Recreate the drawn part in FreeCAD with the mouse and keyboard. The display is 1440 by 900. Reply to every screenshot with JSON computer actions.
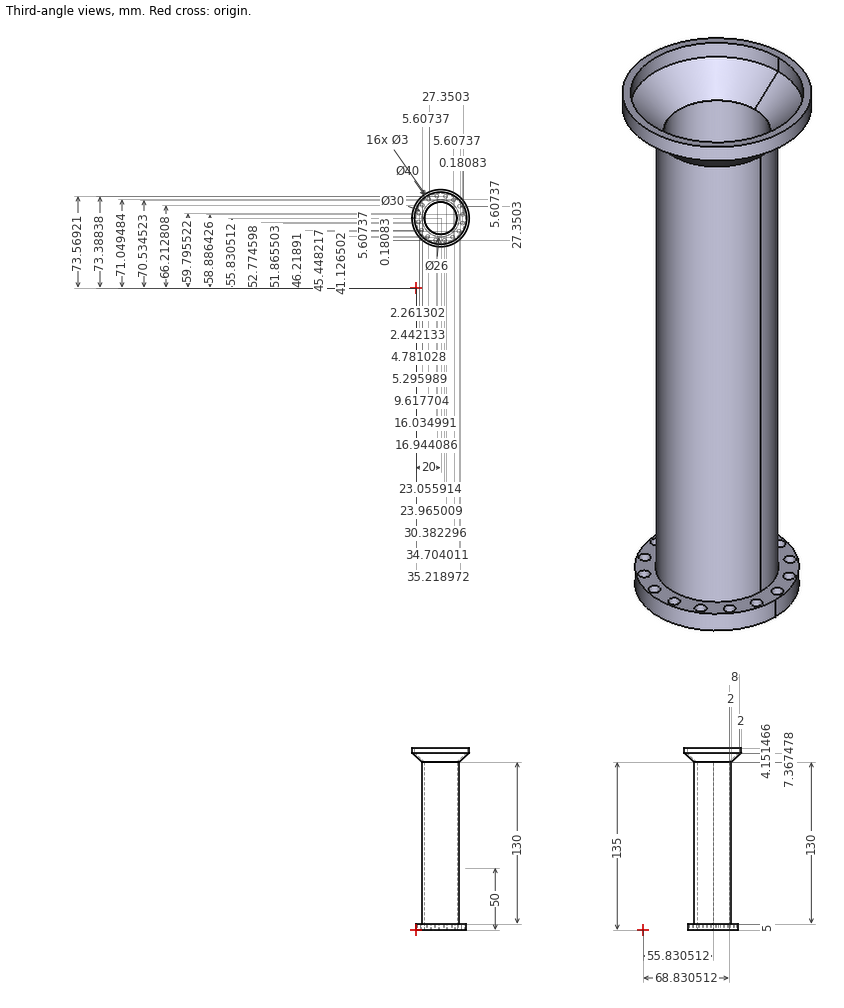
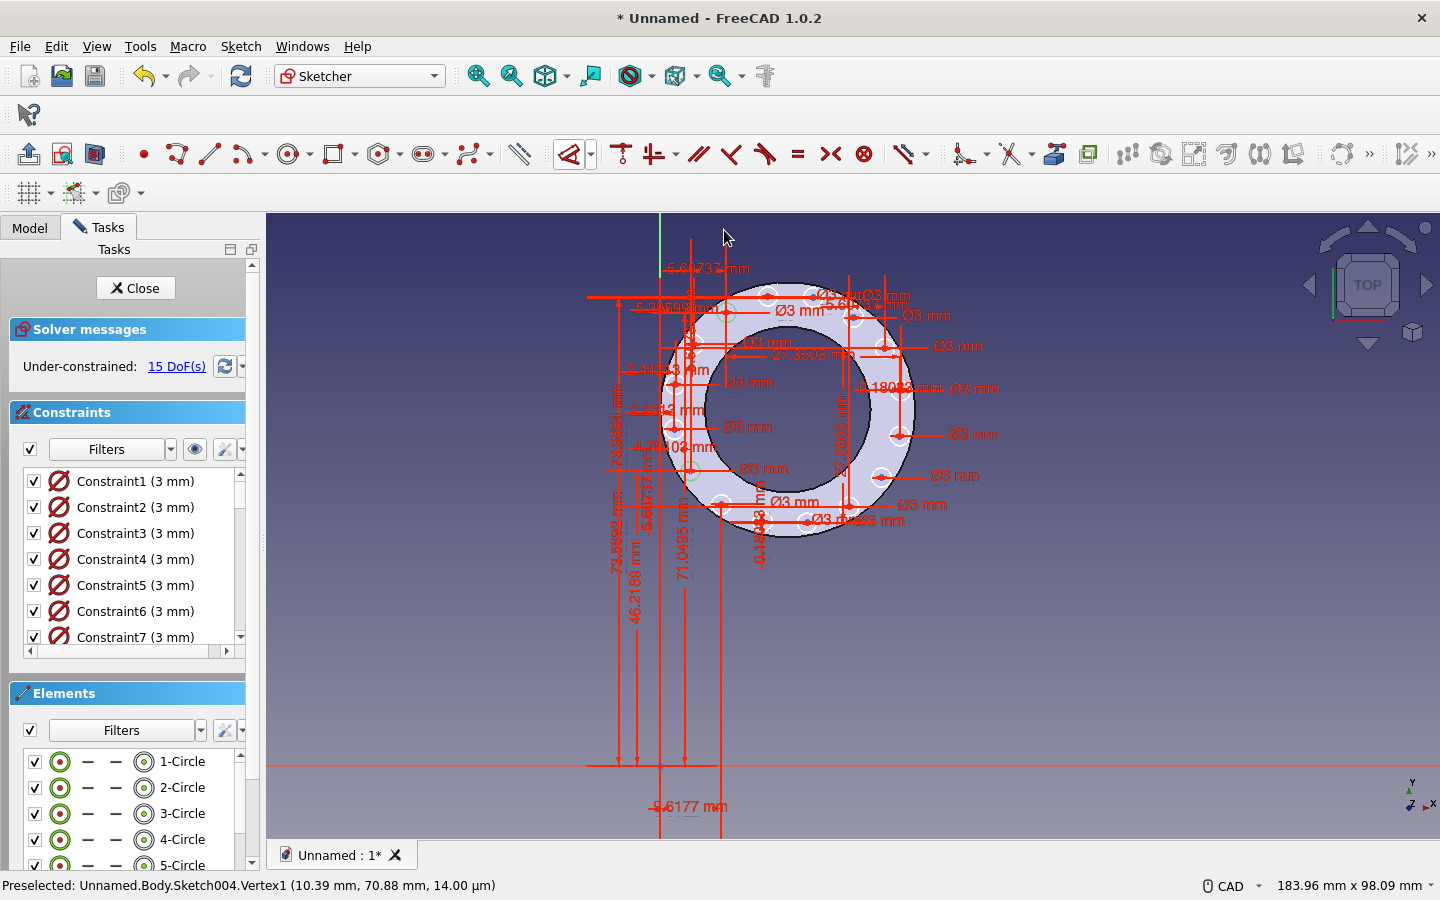
{"action": "left_click", "coordinate": [768, 297]}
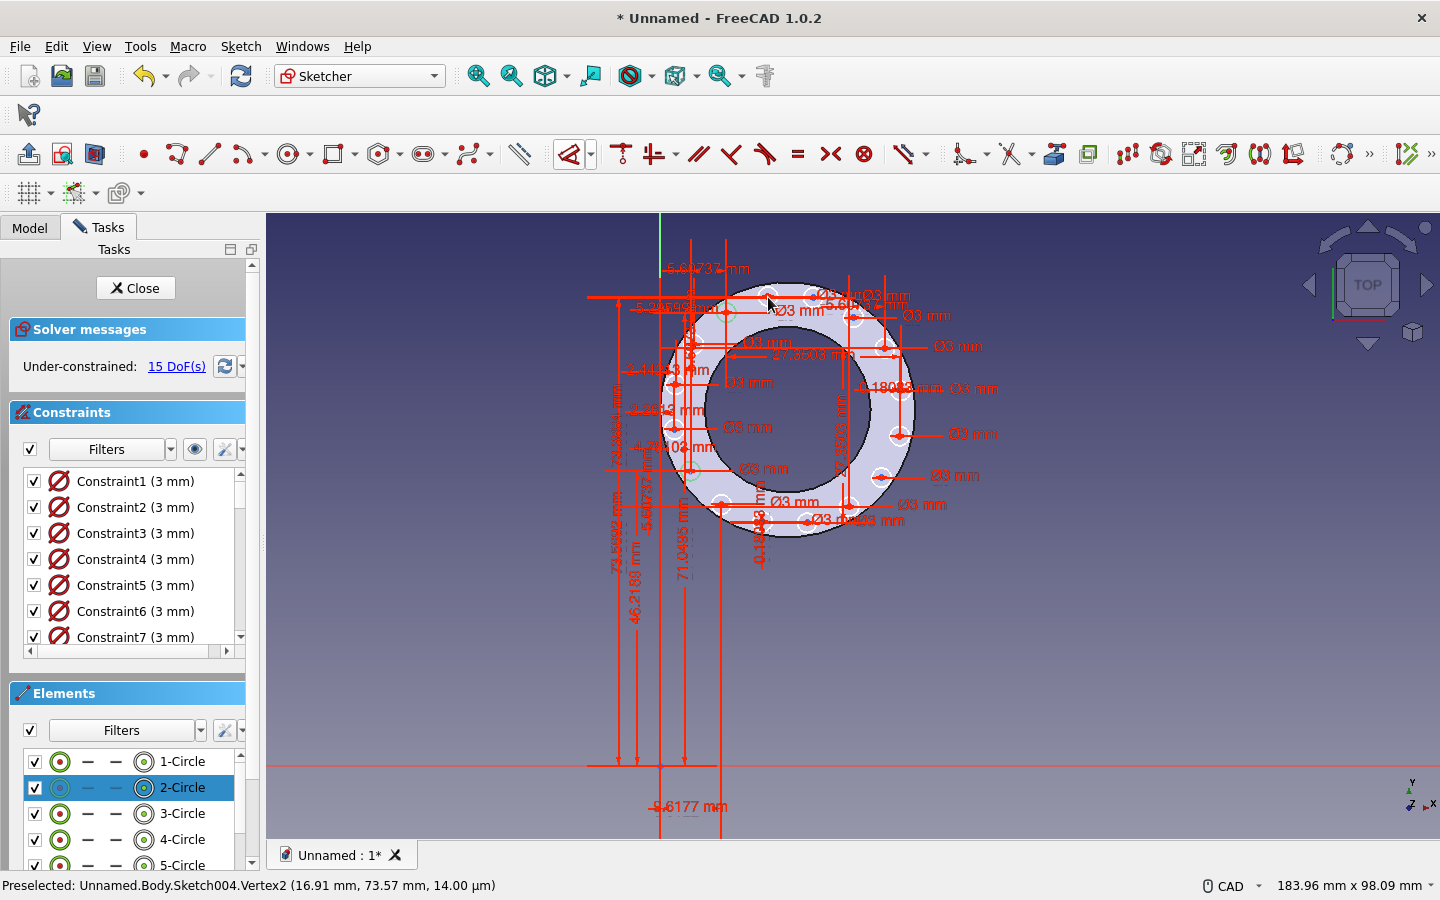
{"action": "left_click", "coordinate": [590, 154]}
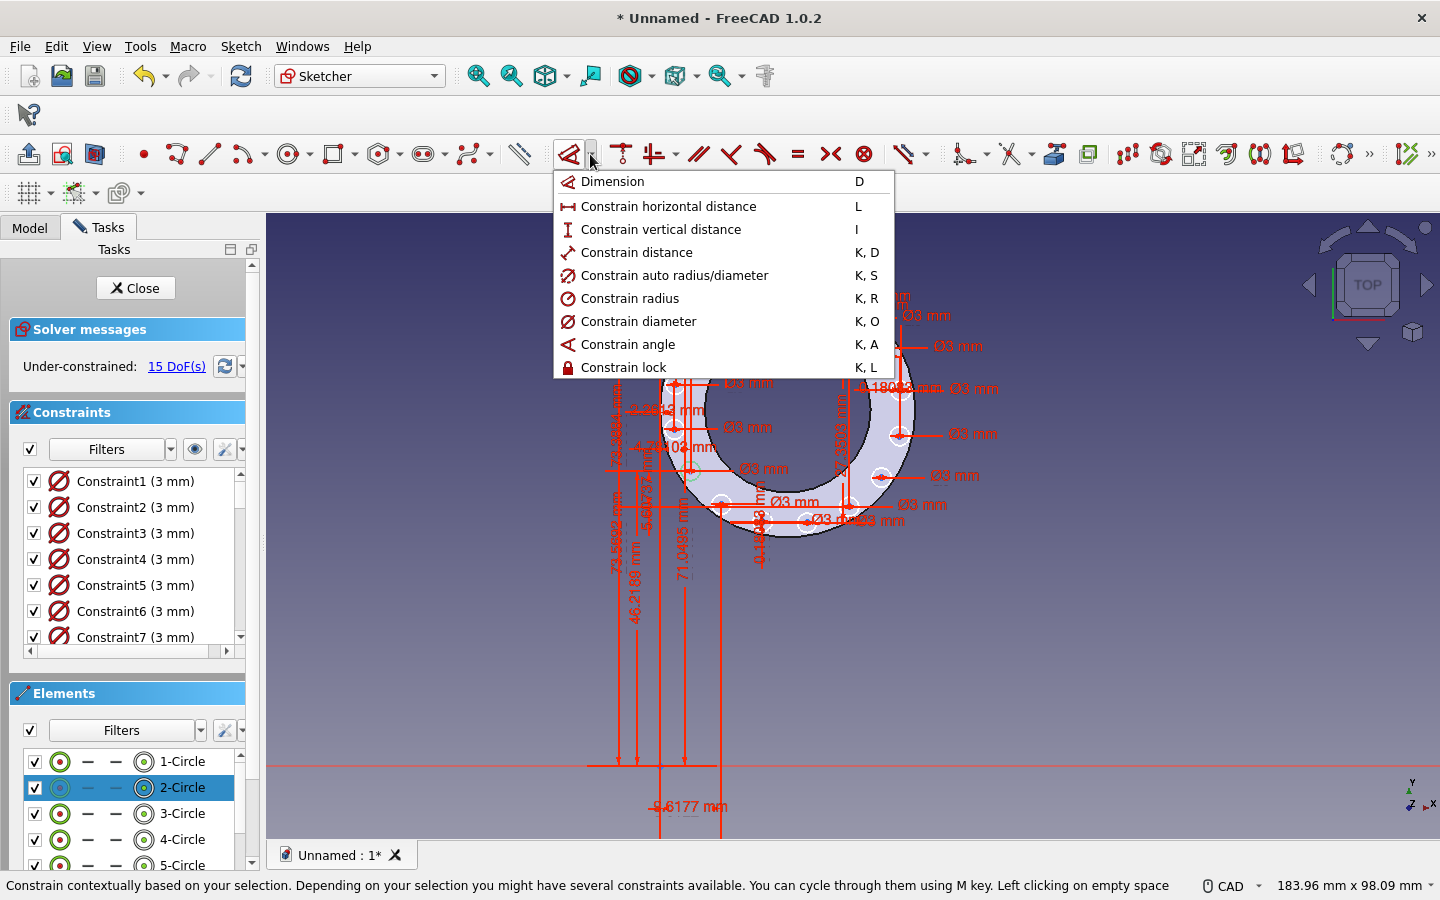
{"action": "left_click", "coordinate": [724, 206]}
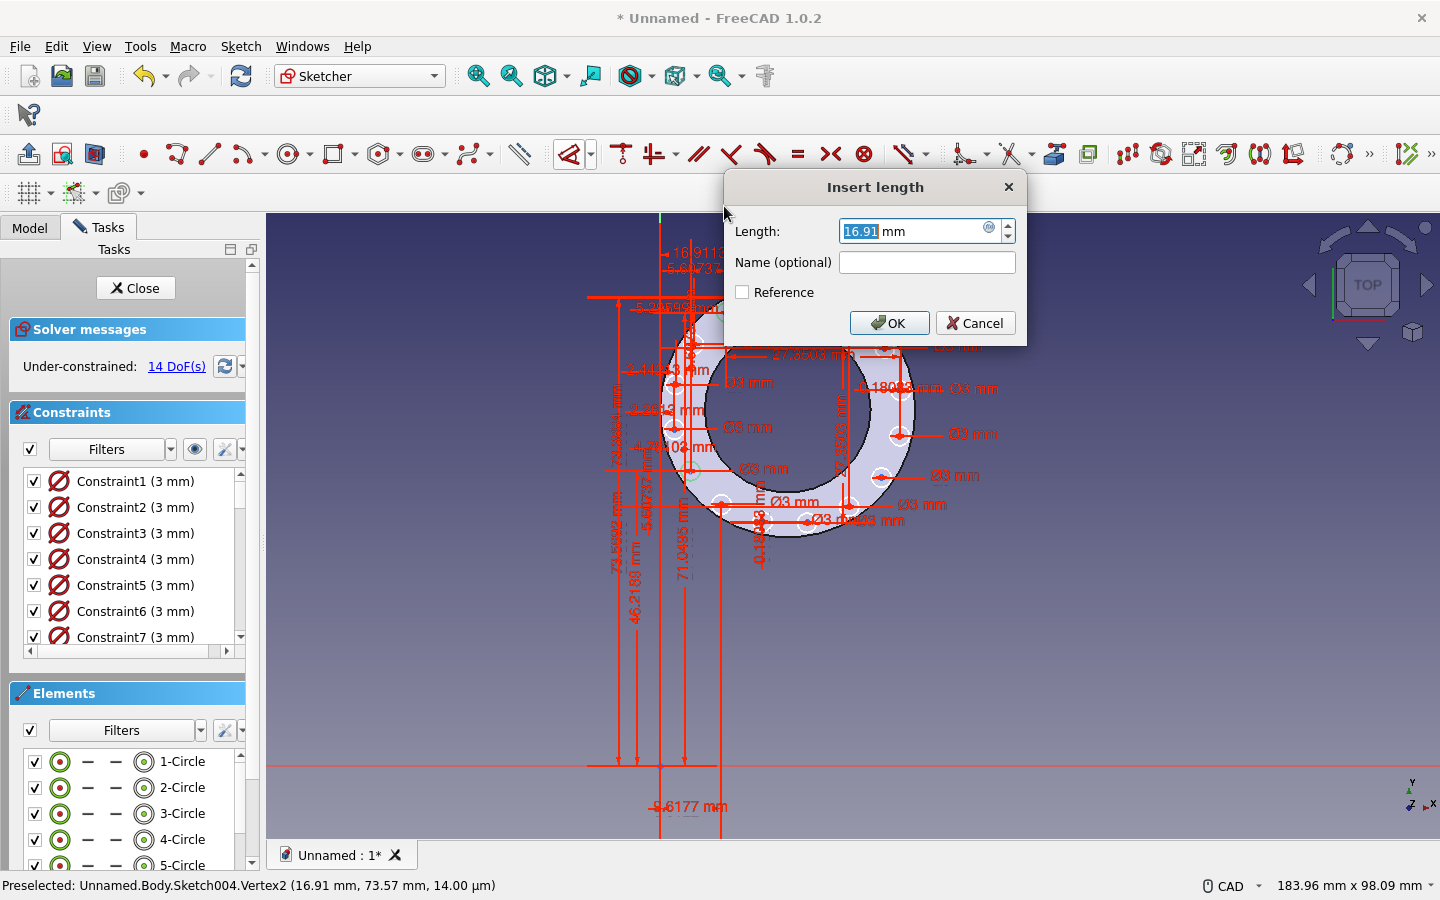
{"action": "type", "text": "16.944086"}
{"action": "key", "text": "Return"}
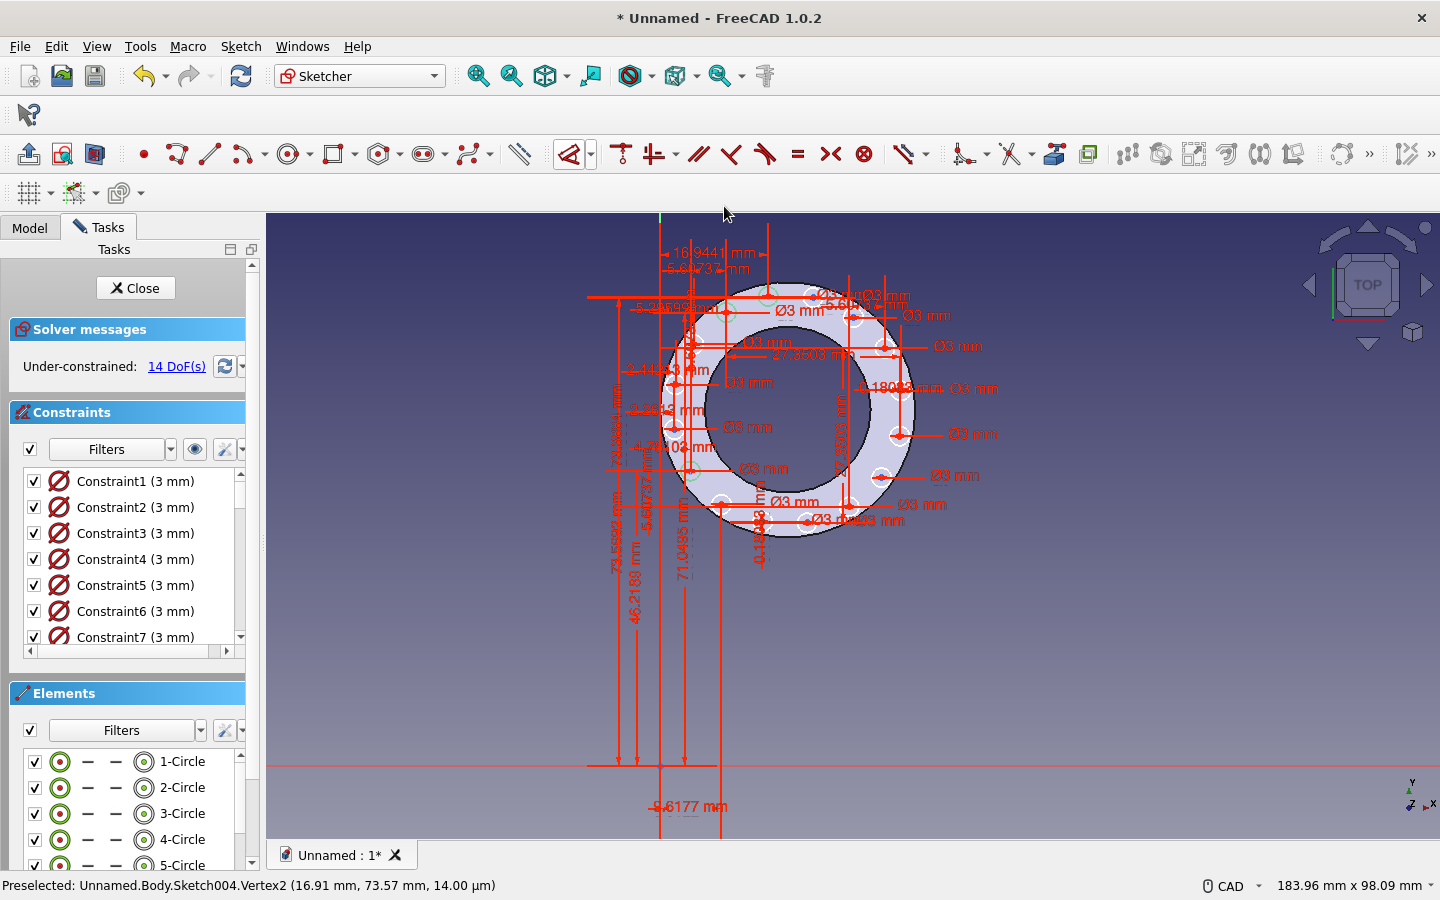
{"action": "left_click", "coordinate": [813, 298]}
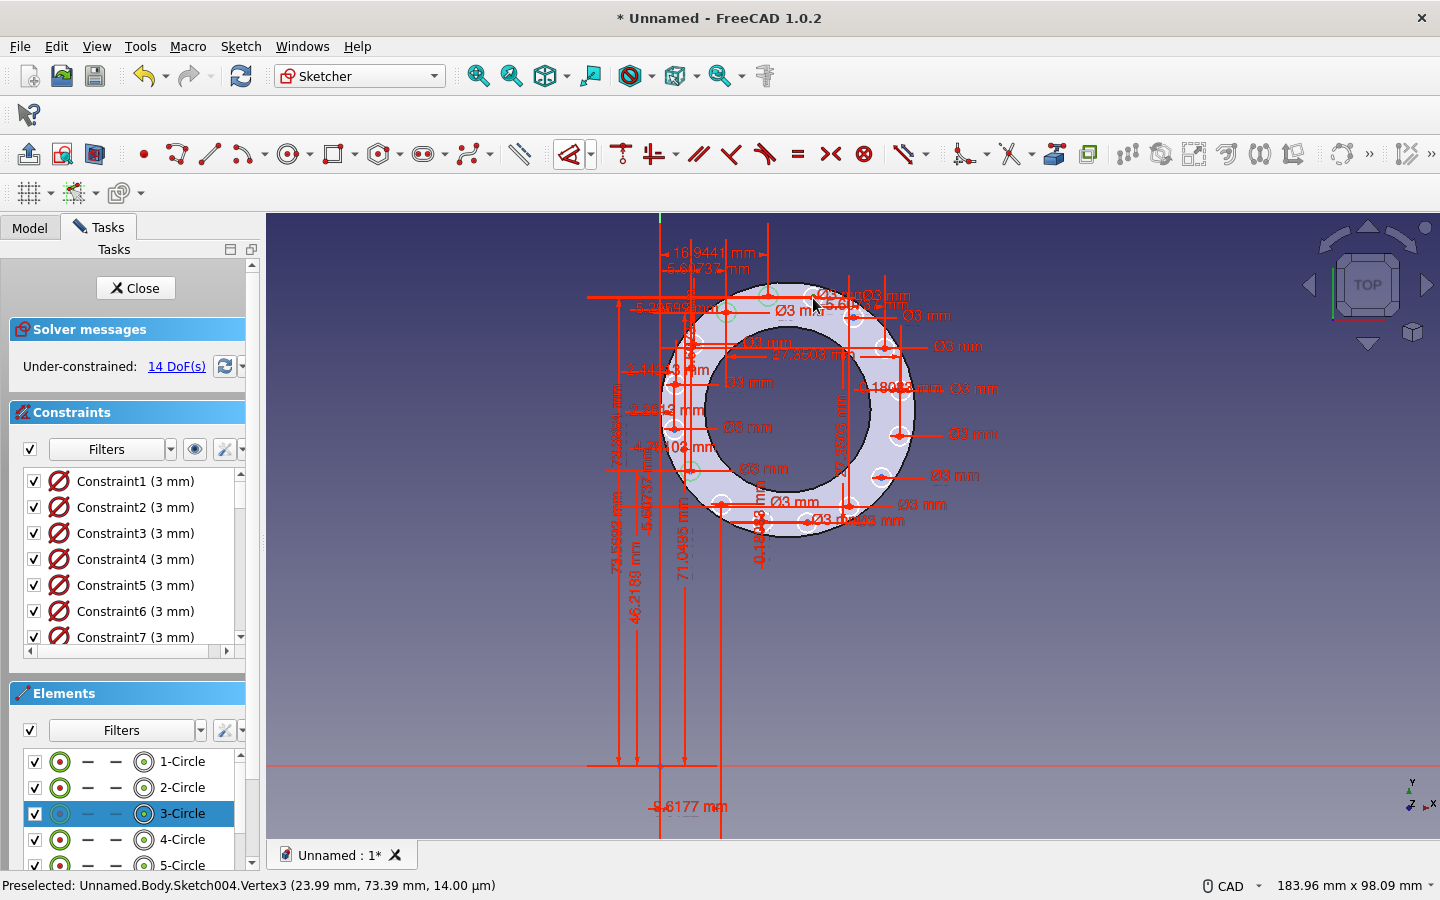
{"action": "left_click", "coordinate": [590, 154]}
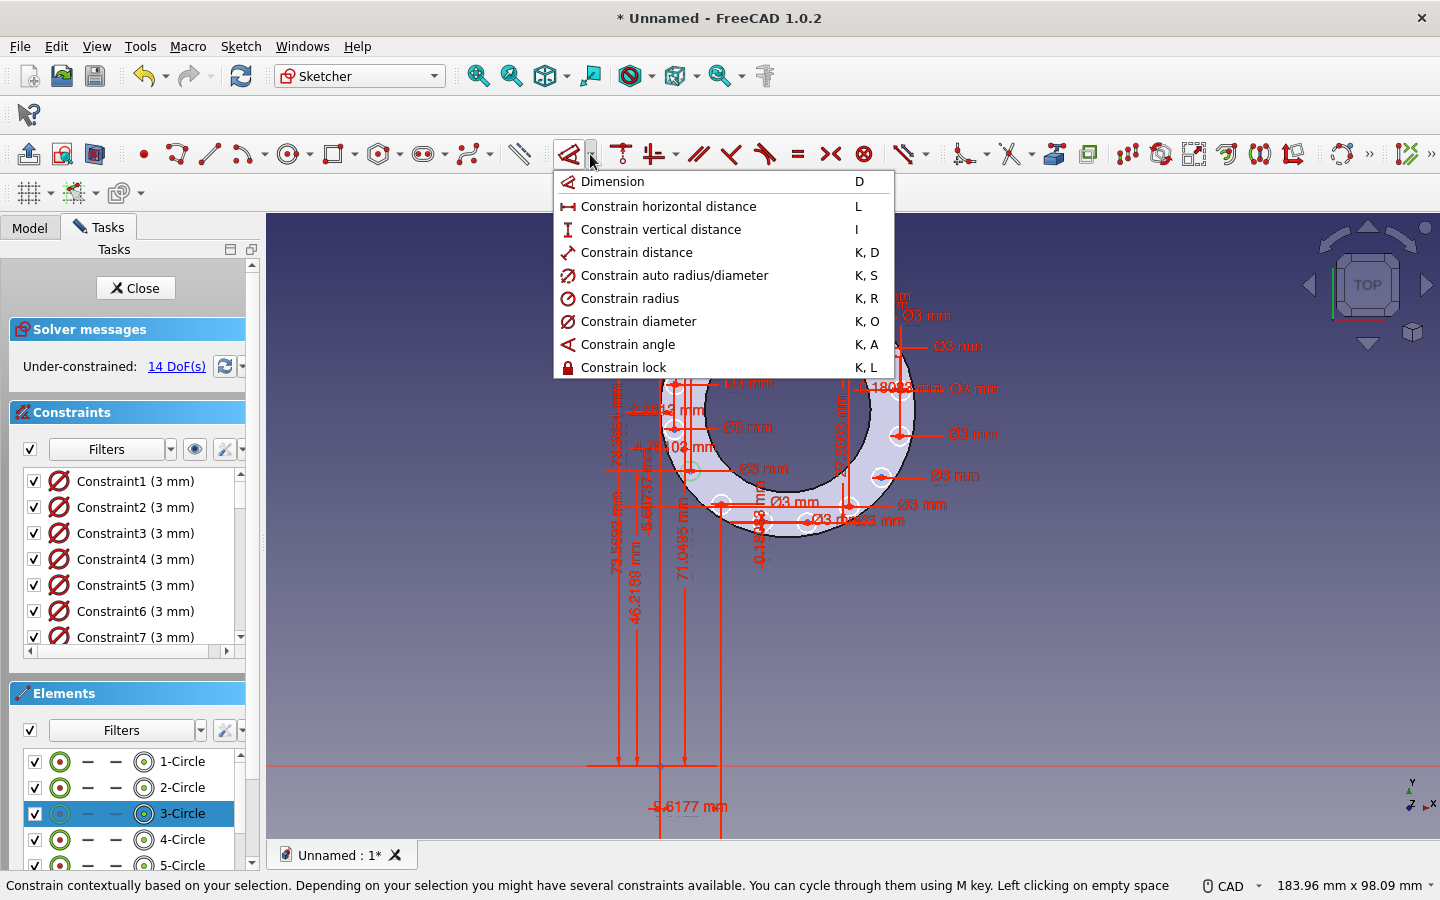
{"action": "left_click", "coordinate": [724, 206]}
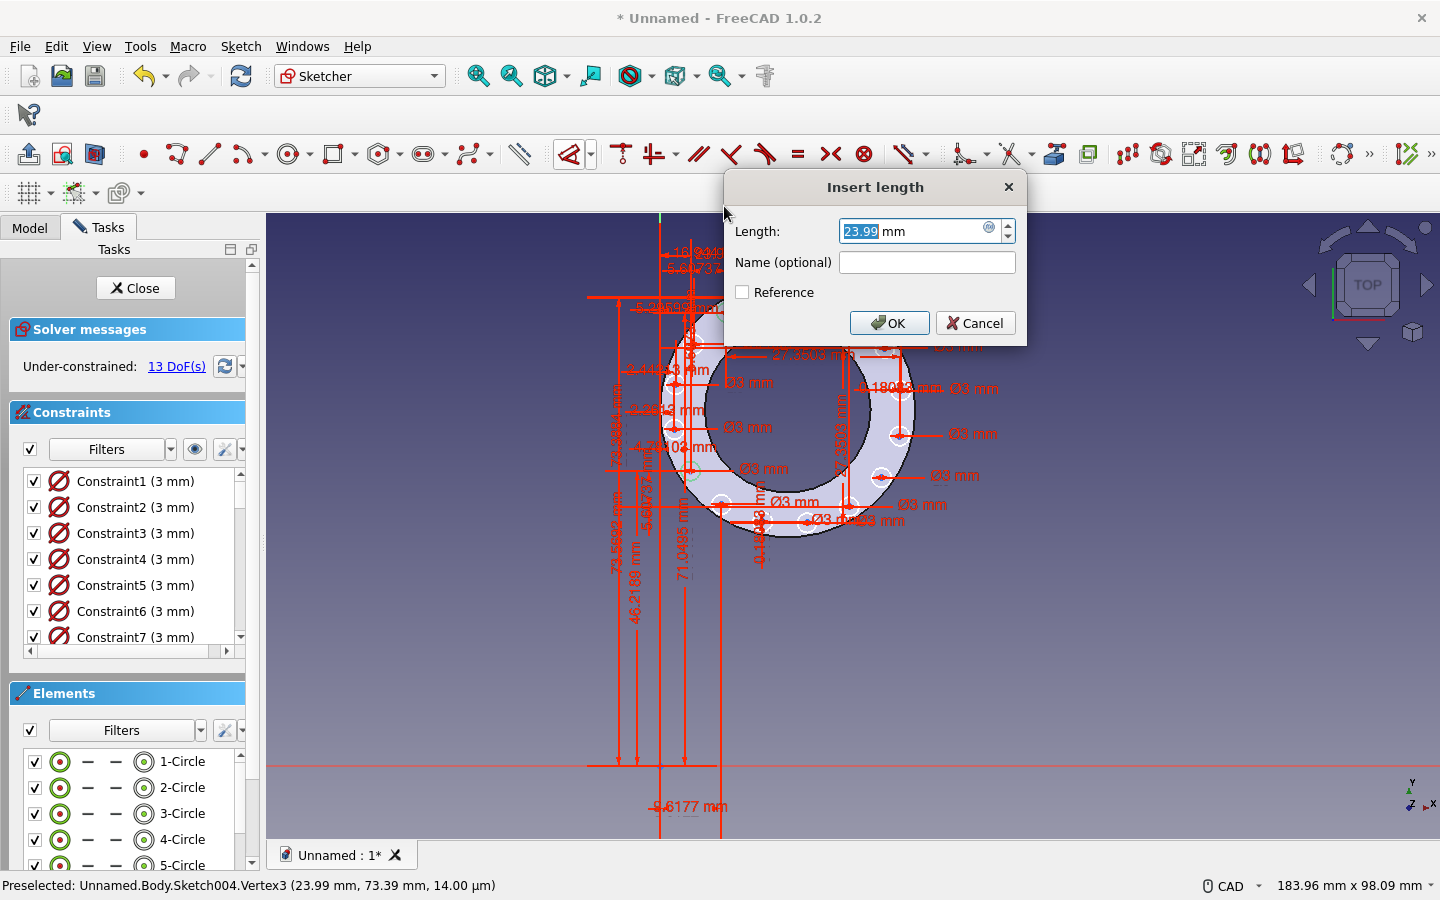
{"action": "type", "text": "23.965009"}
{"action": "key", "text": "Return"}